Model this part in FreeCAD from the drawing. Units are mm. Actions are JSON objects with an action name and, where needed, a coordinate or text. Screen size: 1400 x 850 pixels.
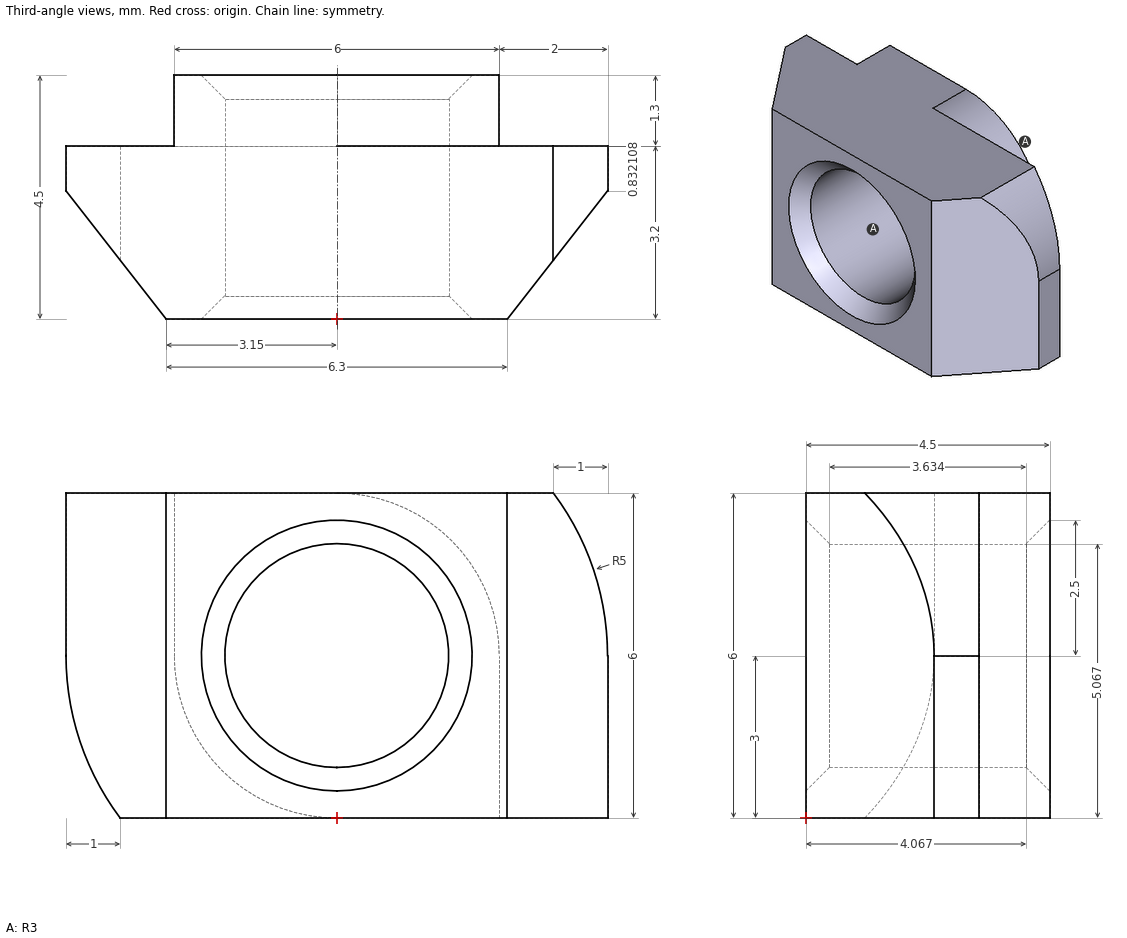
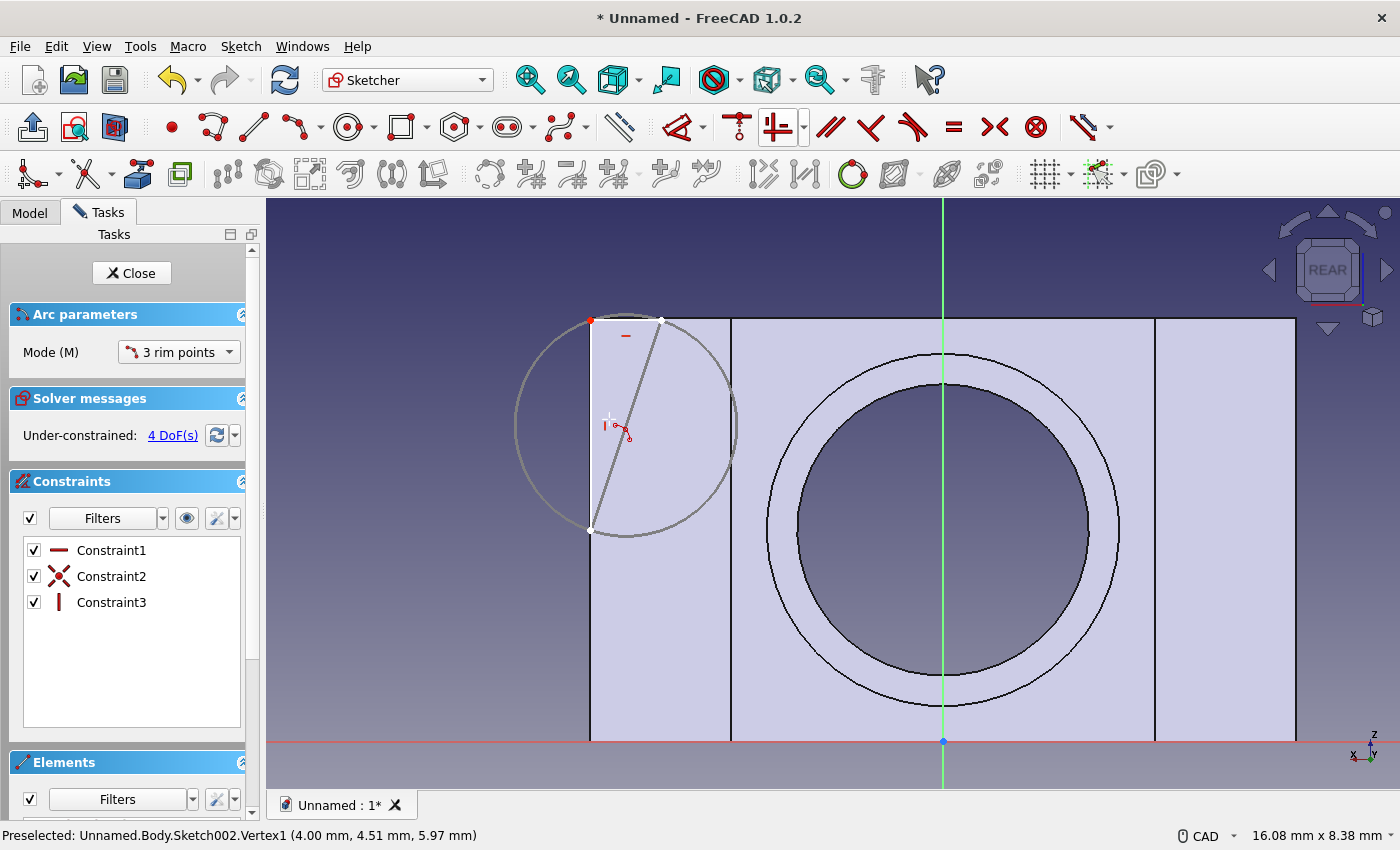
{"action": "left_click", "coordinate": [608, 418]}
{"action": "key", "text": "Escape"}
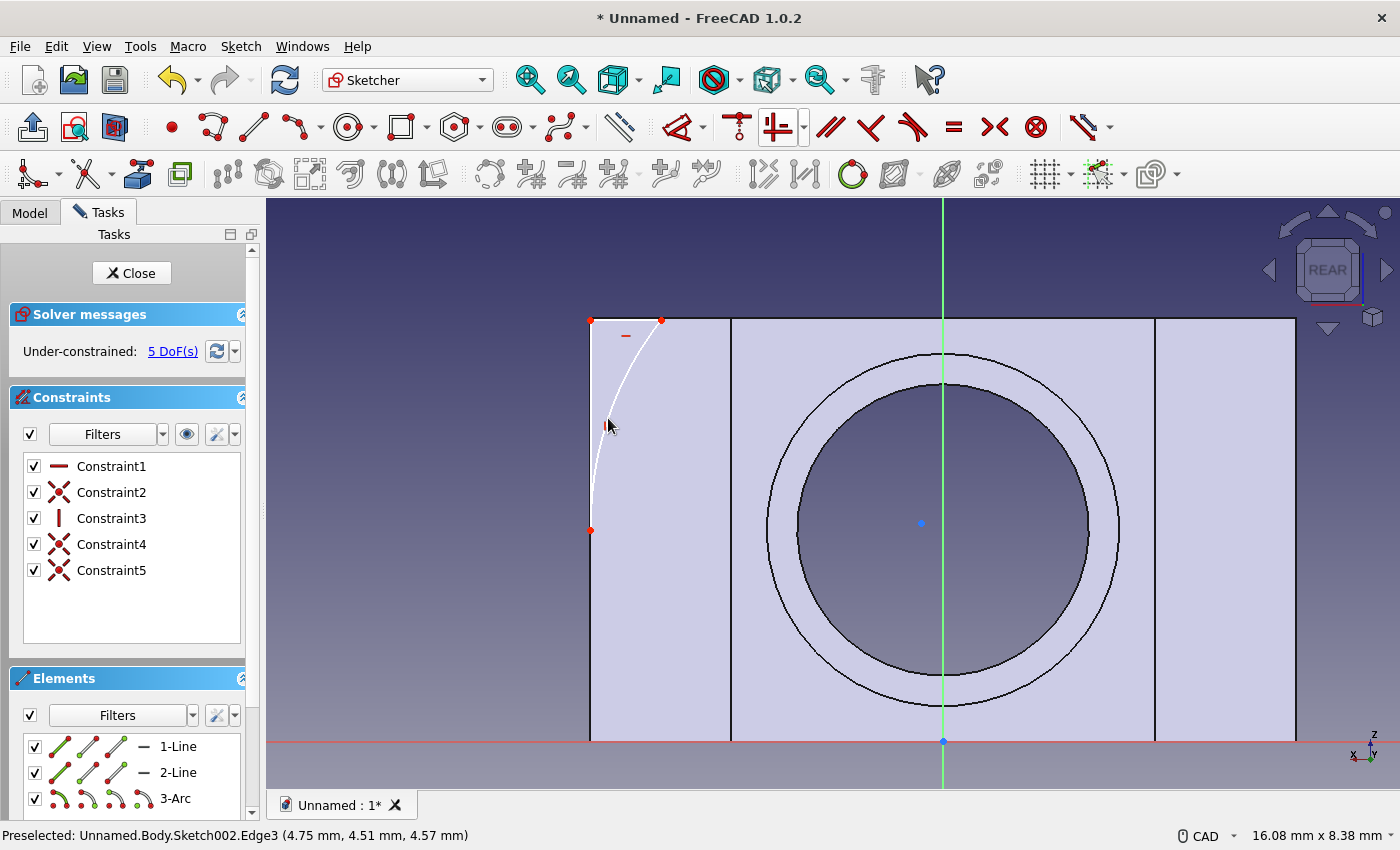
{"action": "left_click", "coordinate": [591, 383]}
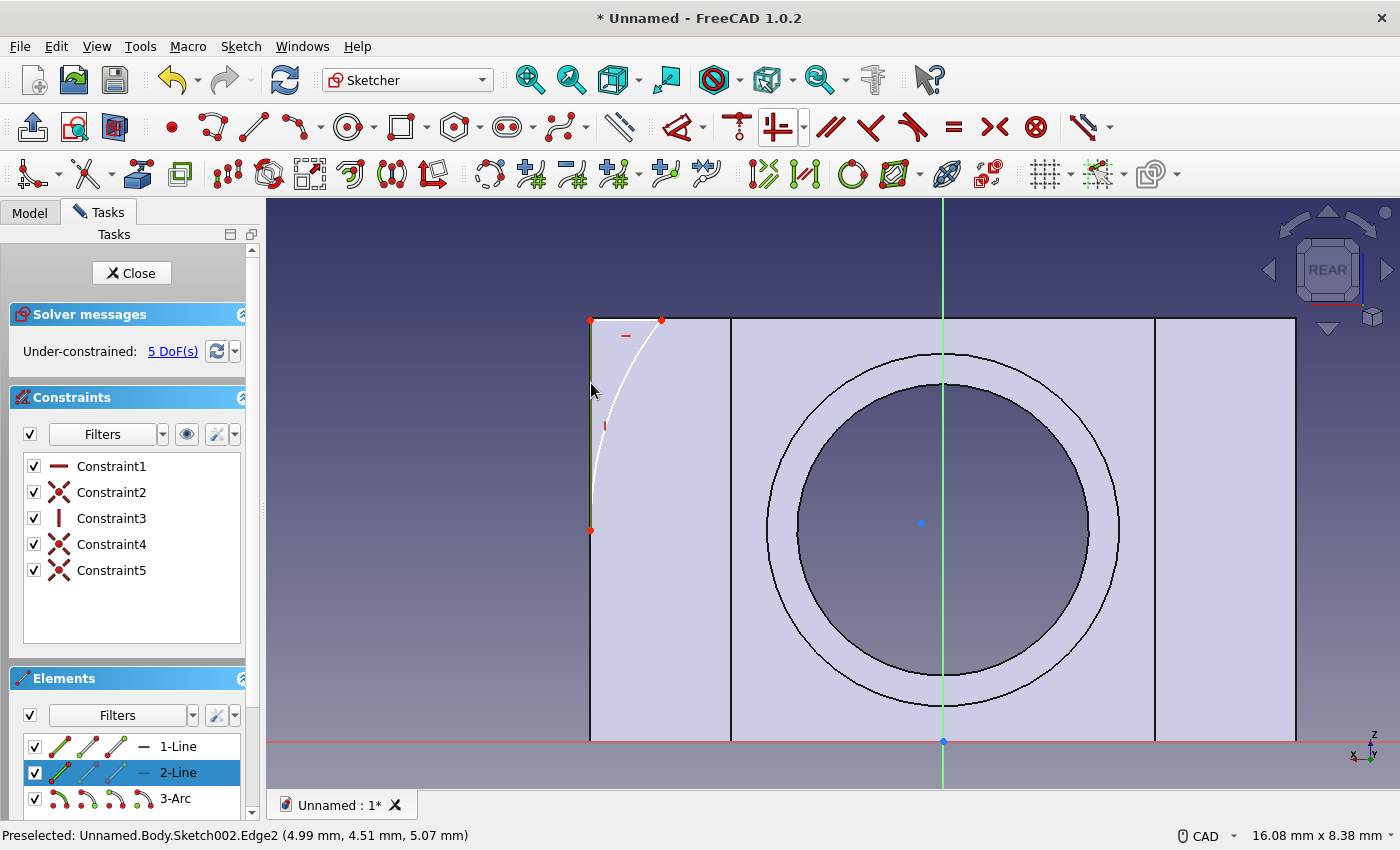
{"action": "left_click", "coordinate": [625, 378]}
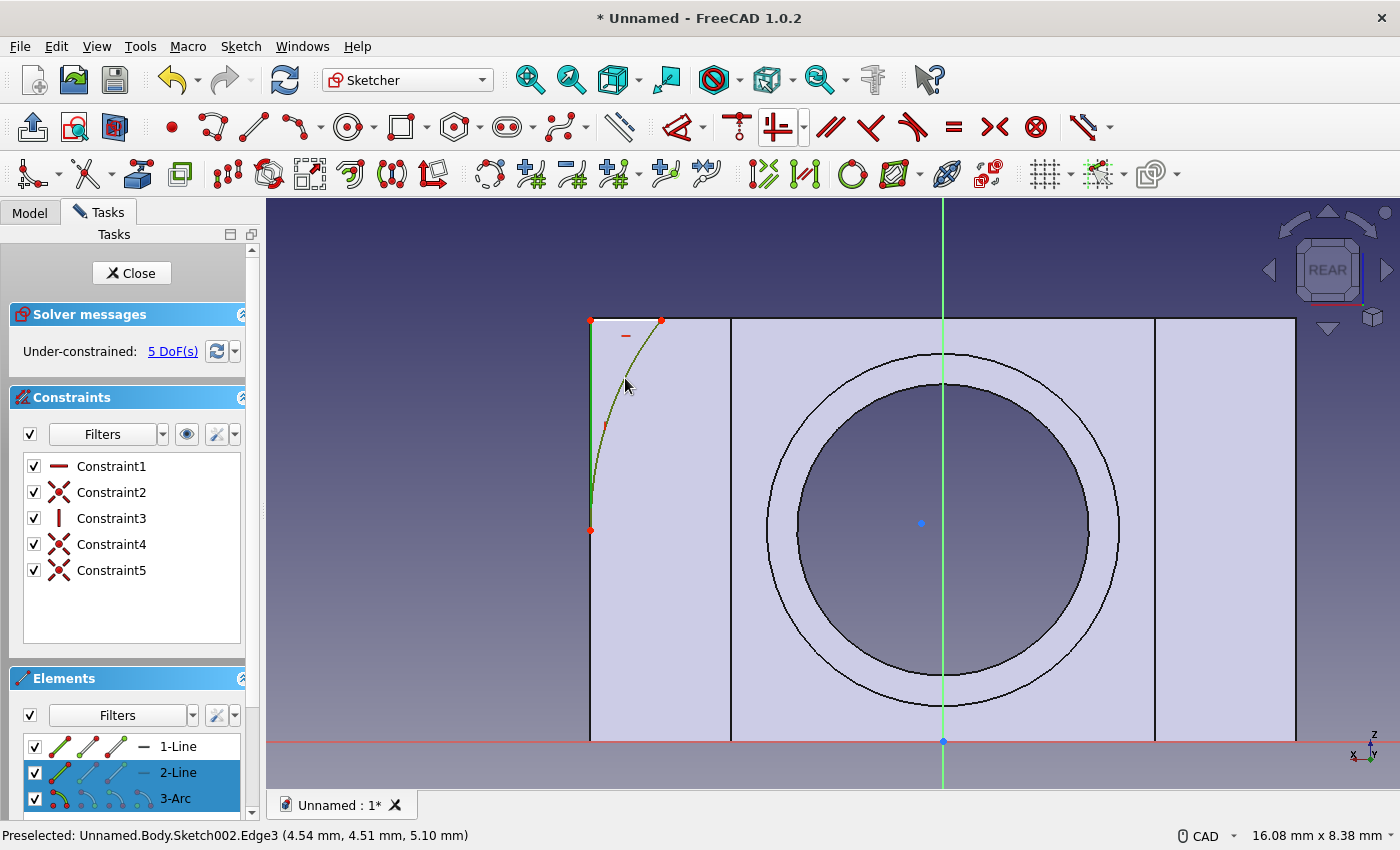
{"action": "left_click", "coordinate": [913, 128]}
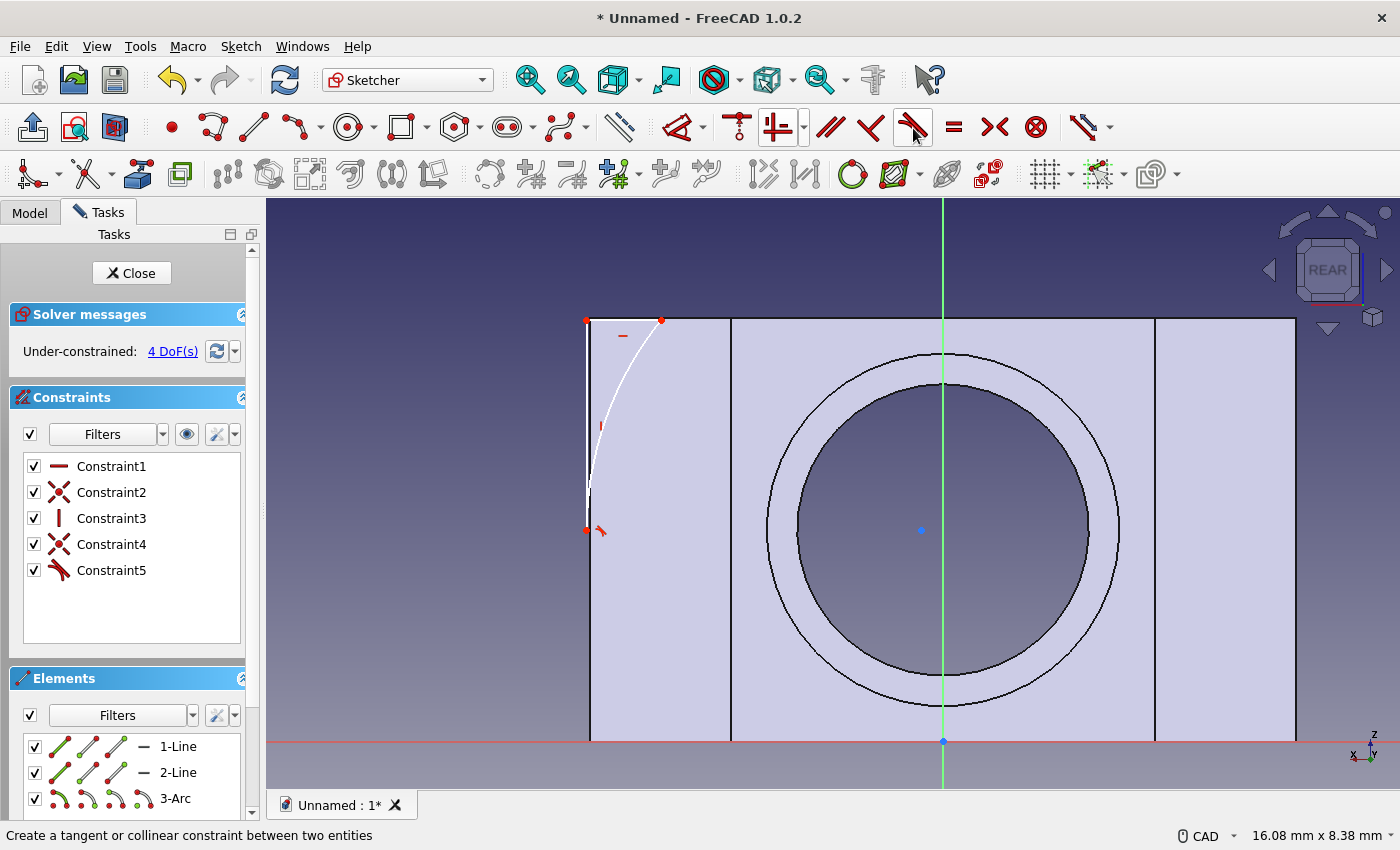
{"action": "left_click", "coordinate": [921, 531]}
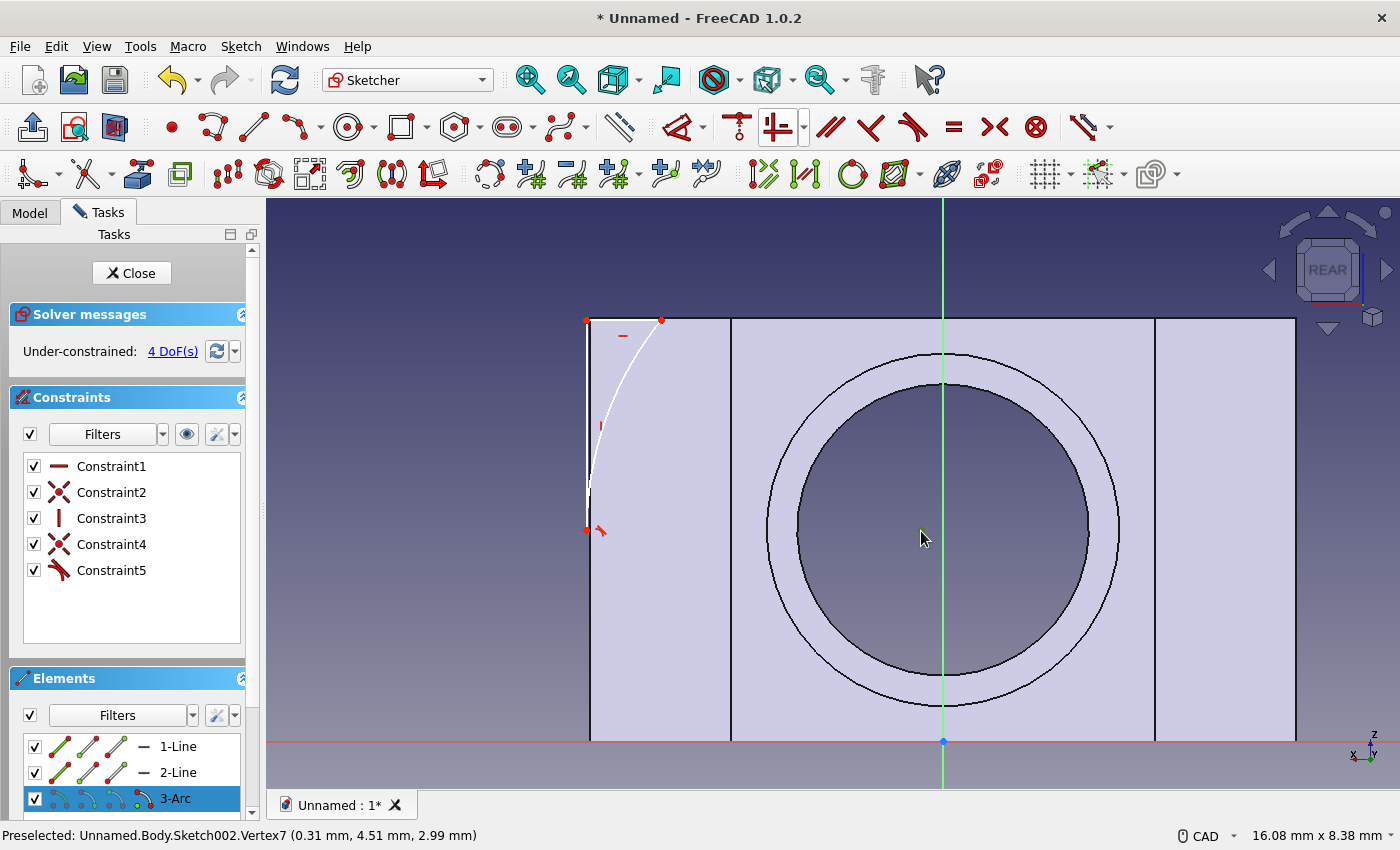
{"action": "left_click", "coordinate": [943, 685]}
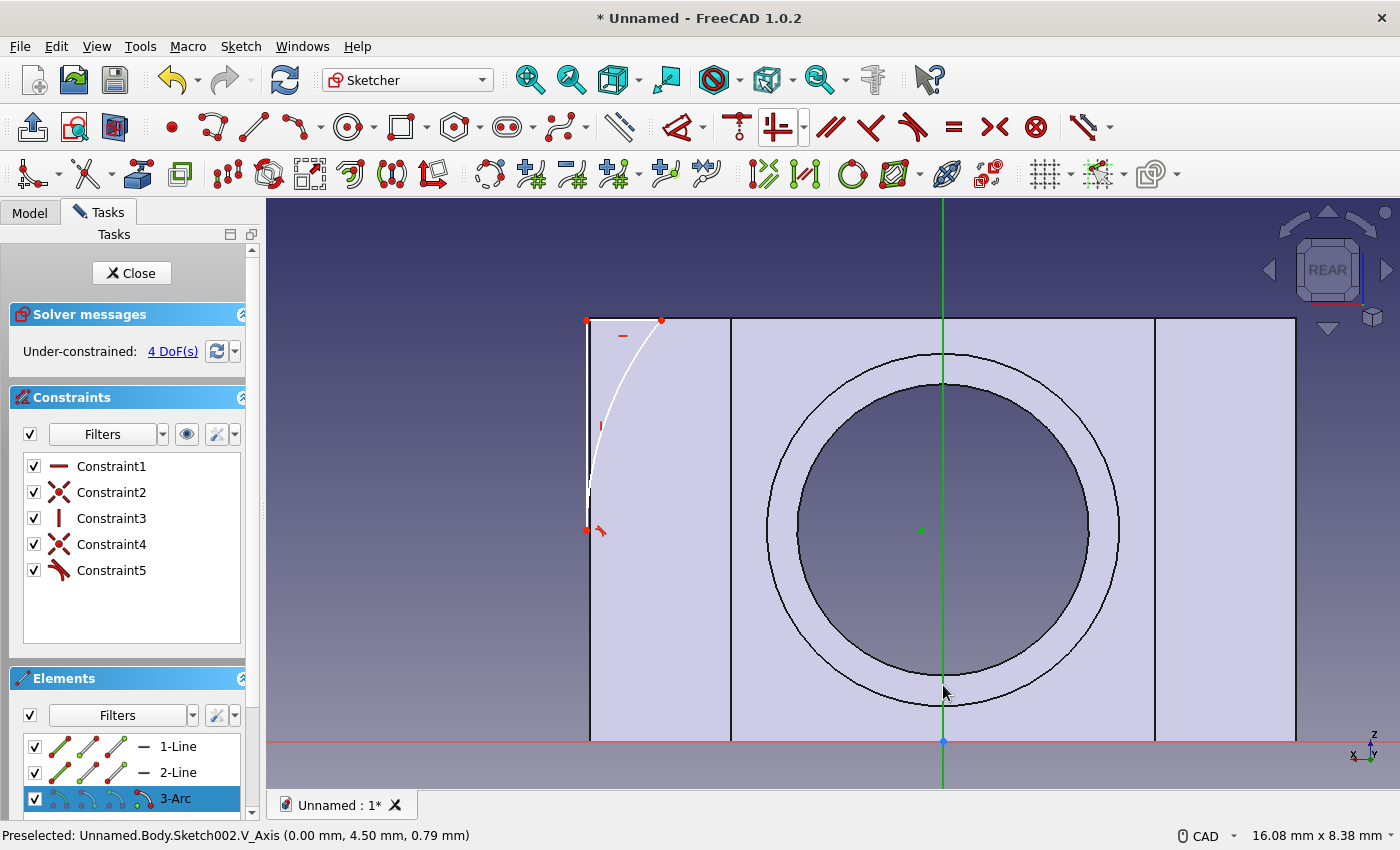
{"action": "left_click", "coordinate": [737, 128]}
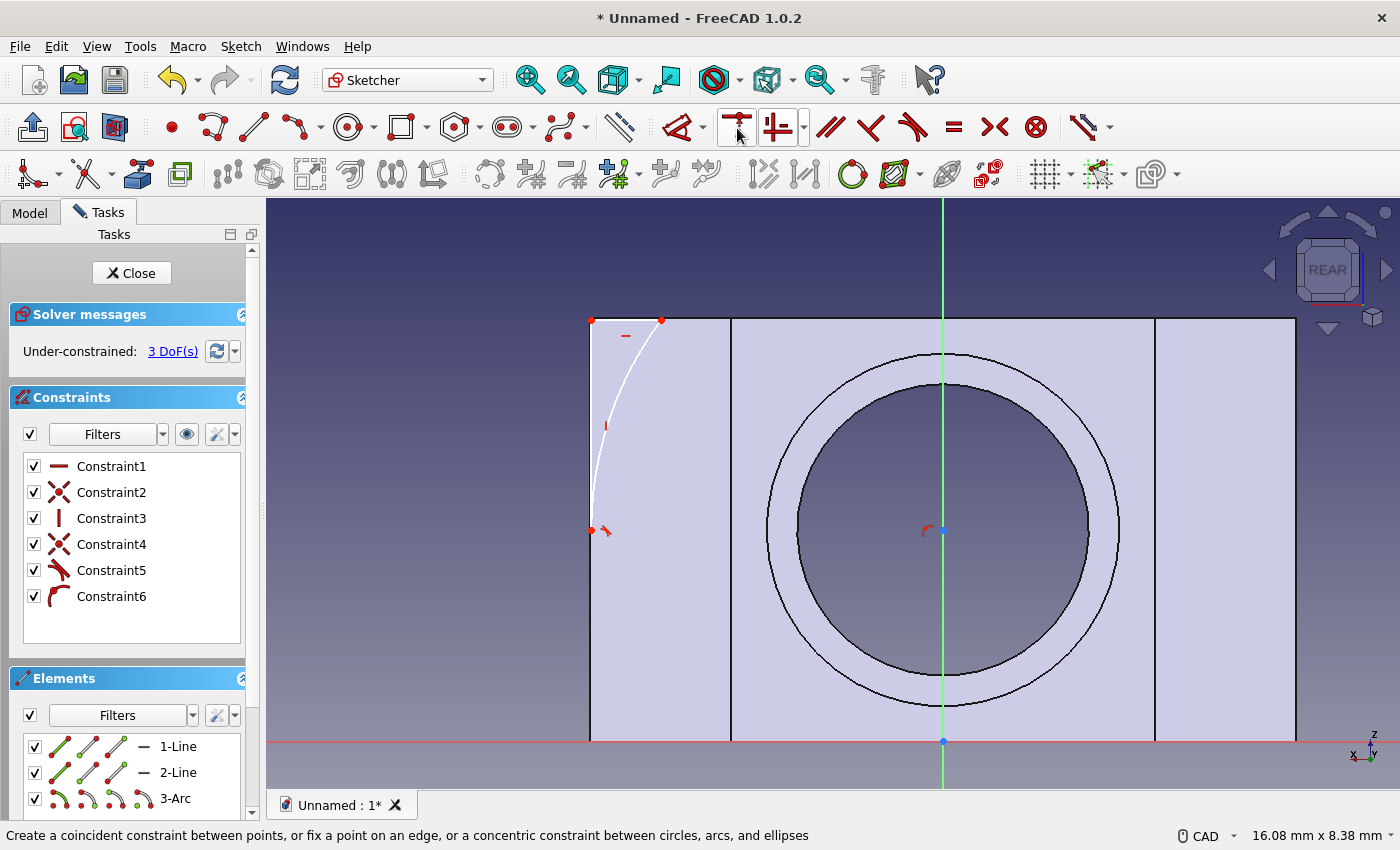
{"action": "left_click", "coordinate": [676, 128]}